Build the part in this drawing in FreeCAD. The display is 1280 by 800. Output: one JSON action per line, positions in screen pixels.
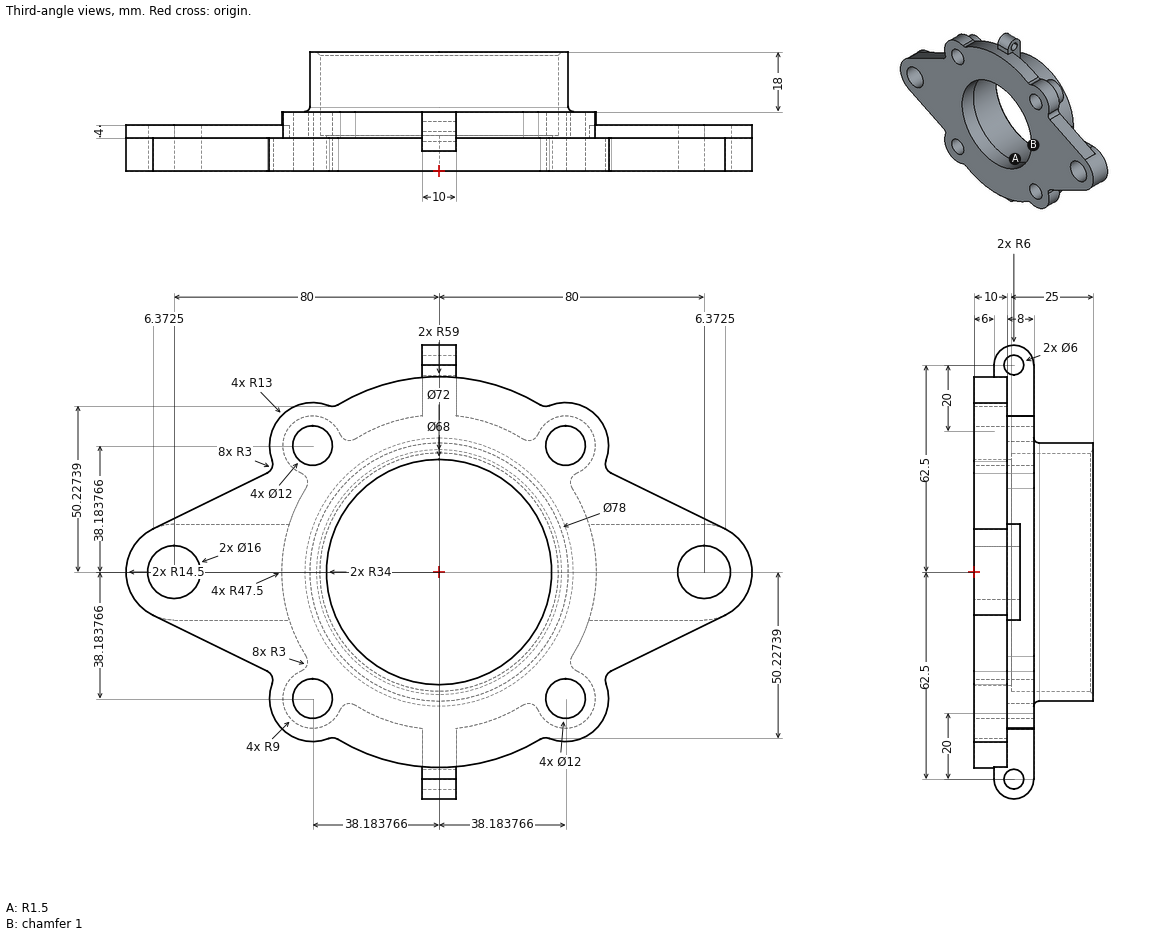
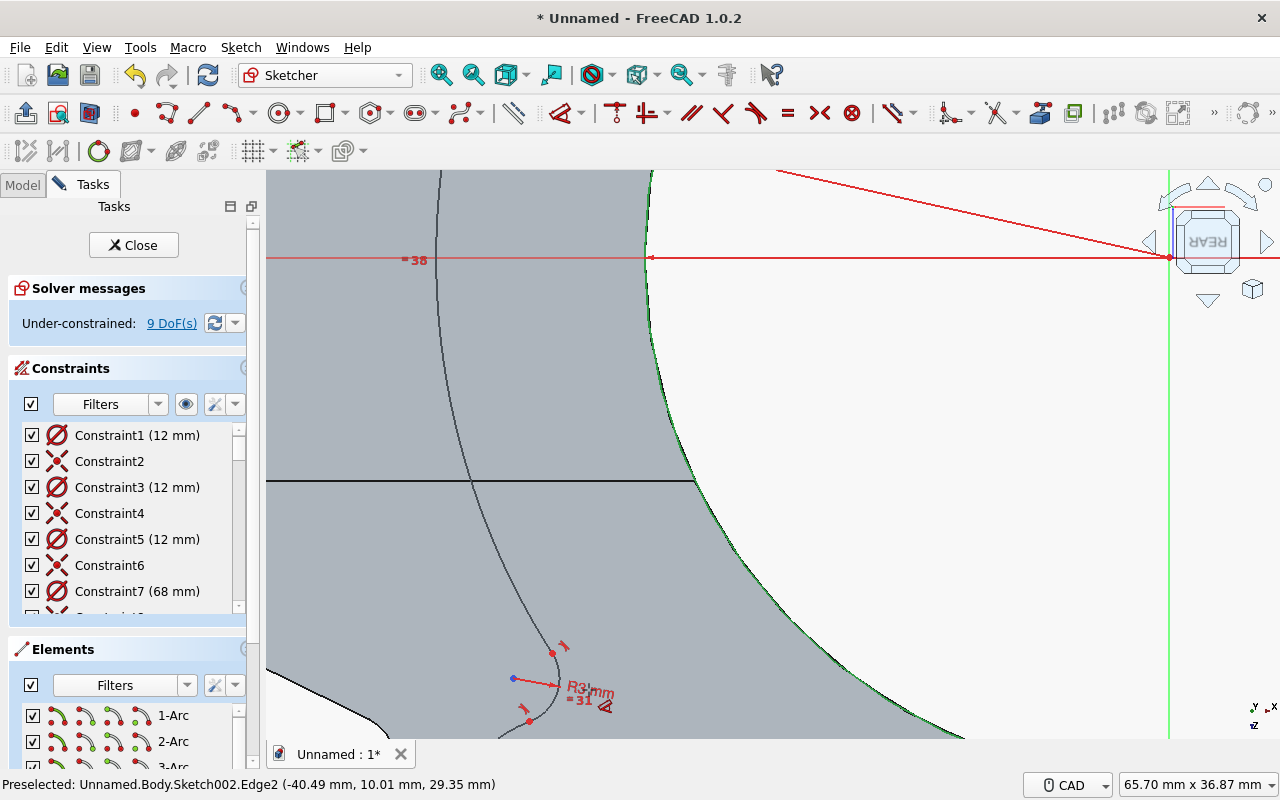
{"action": "scroll", "coordinate": [552, 519], "scroll_direction": "down", "scroll_amount": 7}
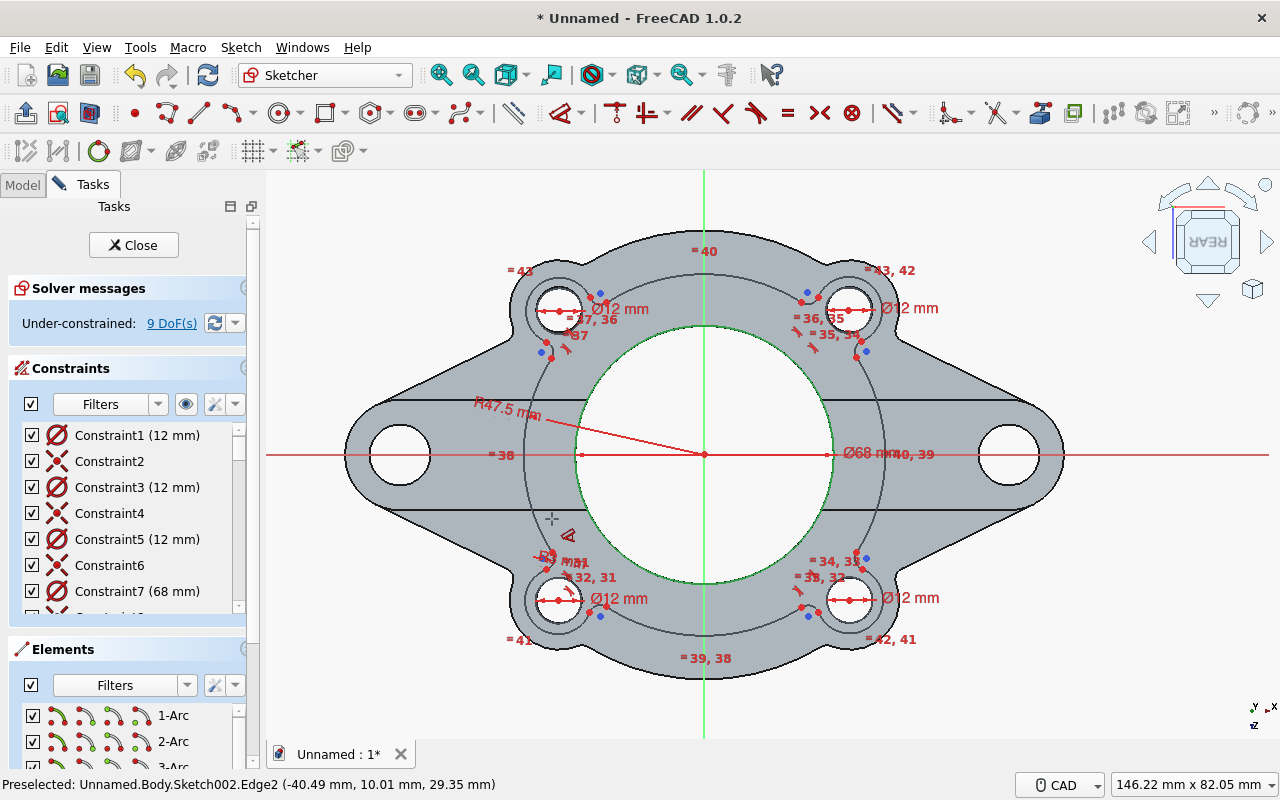
{"action": "scroll", "coordinate": [525, 600], "scroll_direction": "up", "scroll_amount": 2}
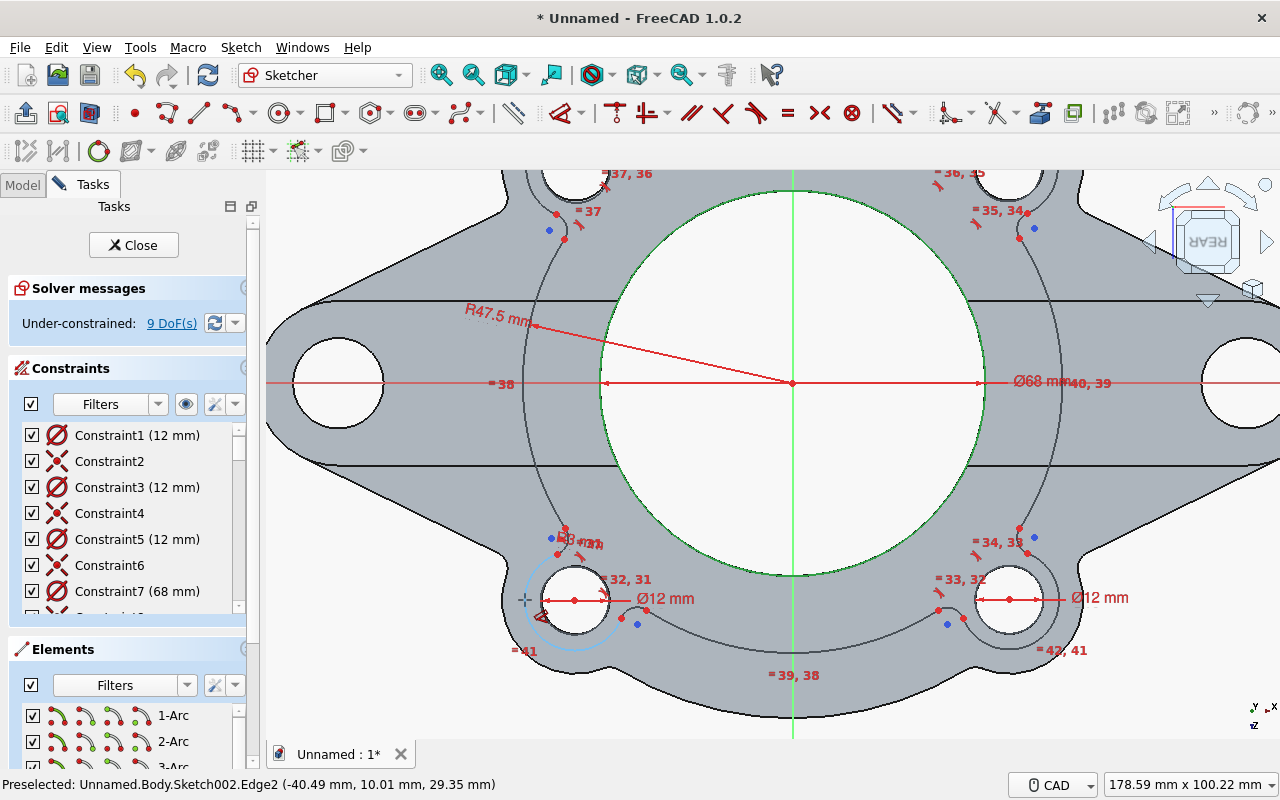
{"action": "left_click", "coordinate": [525, 600]}
{"action": "left_click", "coordinate": [493, 600]}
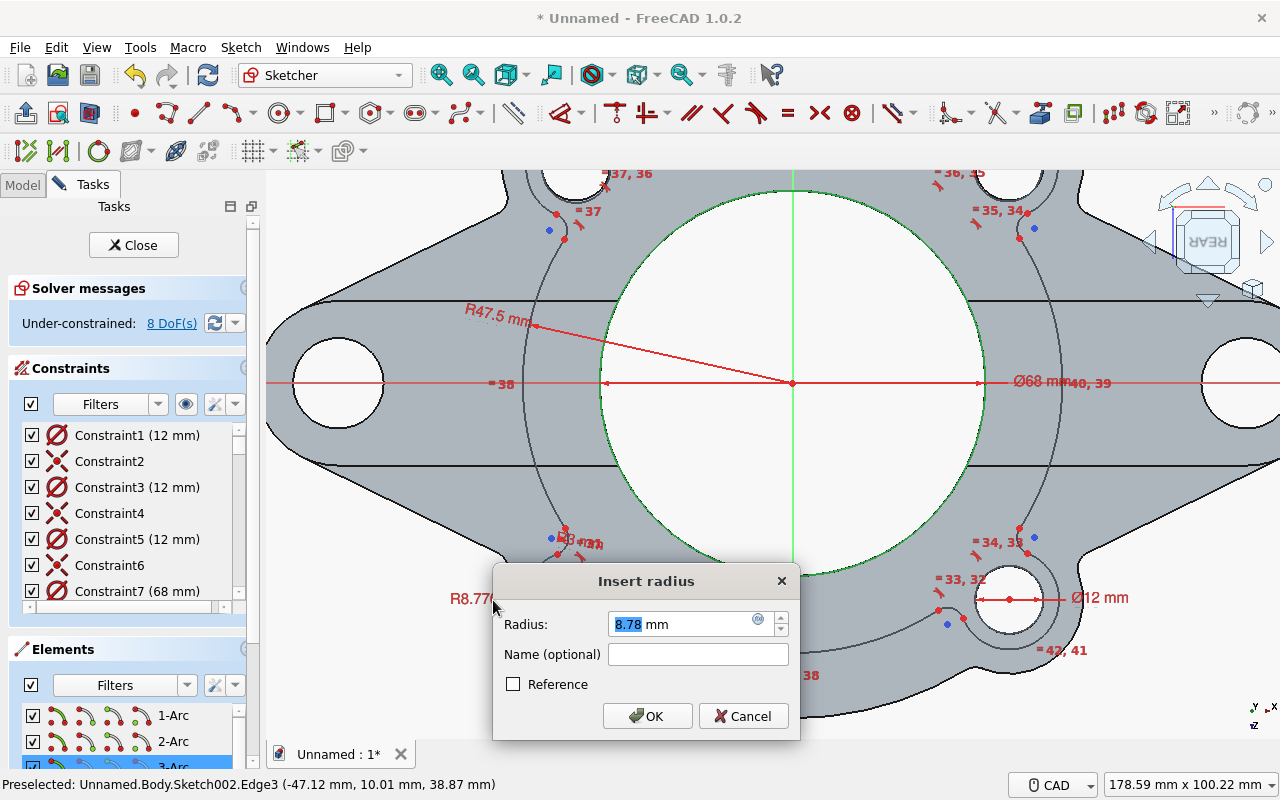
{"action": "type", "text": "9"}
{"action": "key", "text": "Return"}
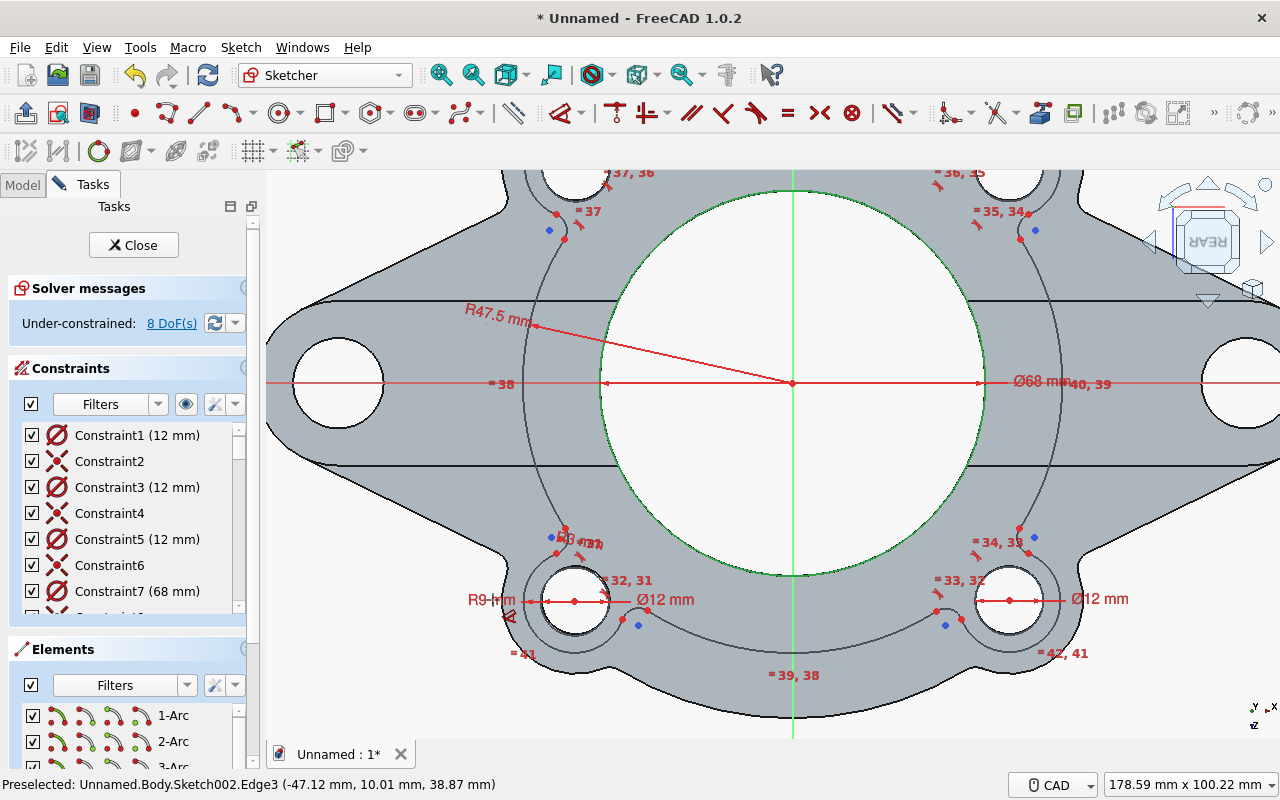
{"action": "left_click", "coordinate": [575, 602]}
{"action": "left_click", "coordinate": [634, 636]}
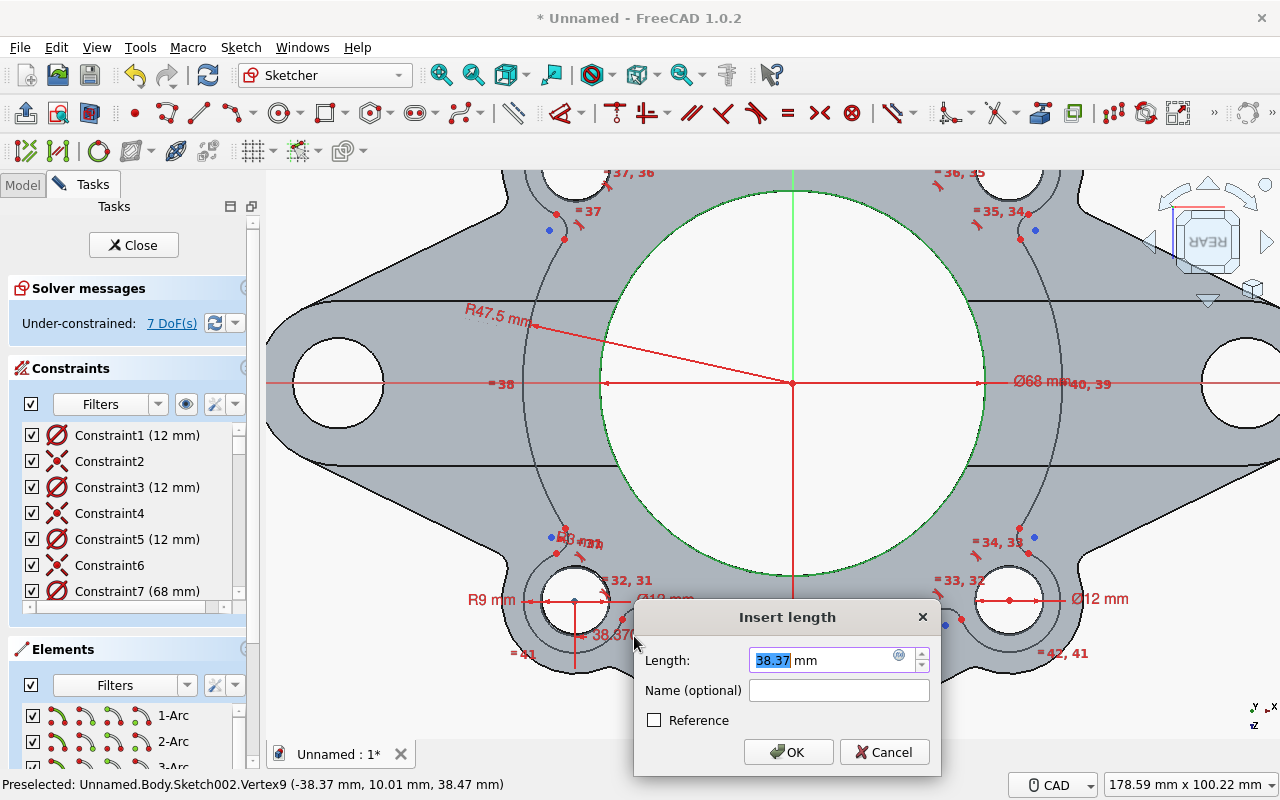
{"action": "type", "text": "38.183766"}
{"action": "key", "text": "Return"}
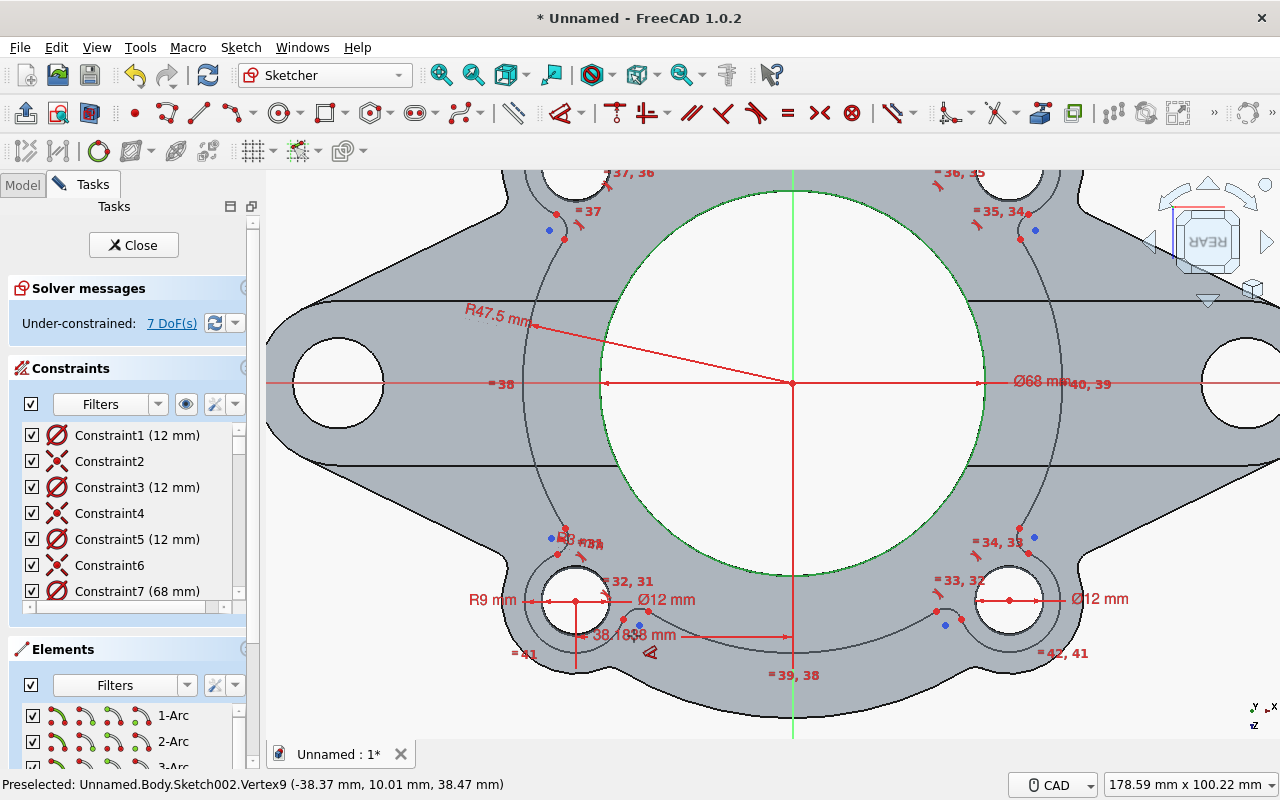
{"action": "left_click", "coordinate": [576, 602]}
{"action": "left_click", "coordinate": [542, 416]}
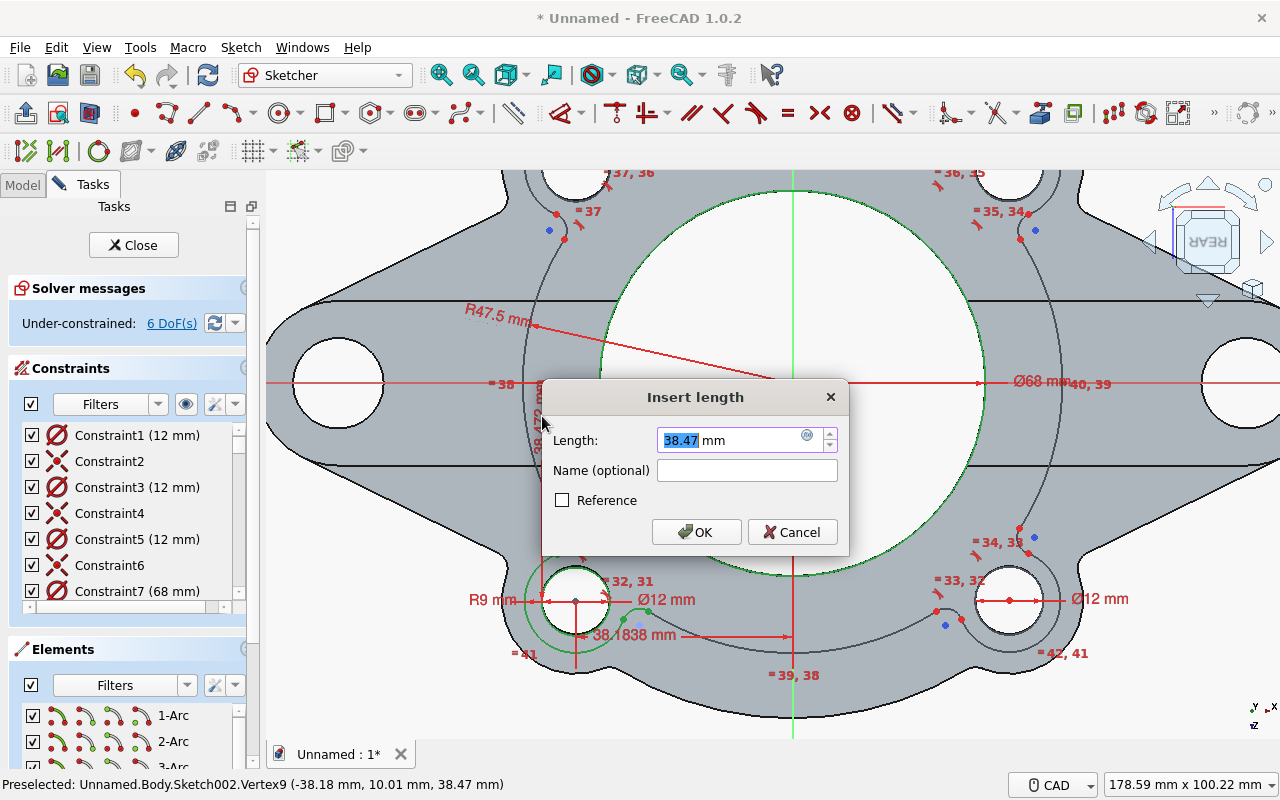
{"action": "type", "text": "38.183766"}
{"action": "key", "text": "Return"}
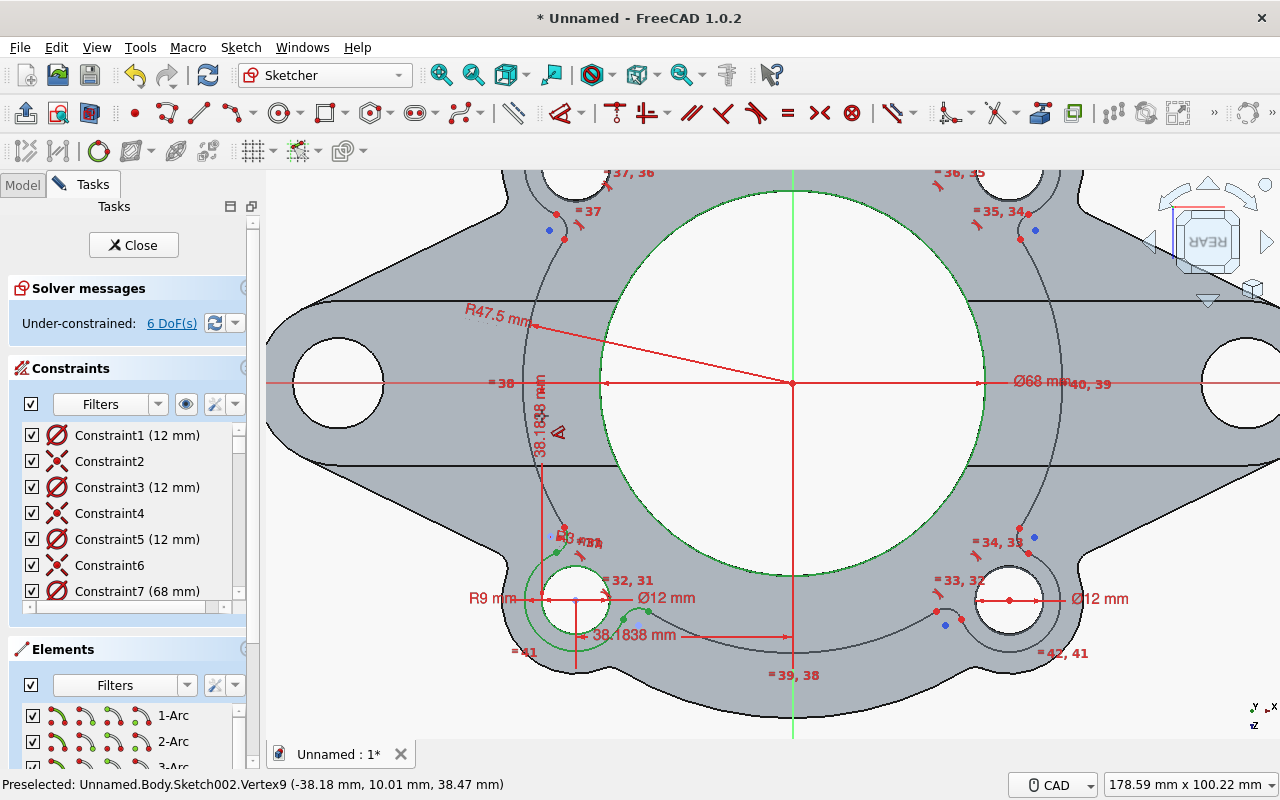
{"action": "left_click", "coordinate": [1009, 601]}
{"action": "left_click", "coordinate": [951, 635]}